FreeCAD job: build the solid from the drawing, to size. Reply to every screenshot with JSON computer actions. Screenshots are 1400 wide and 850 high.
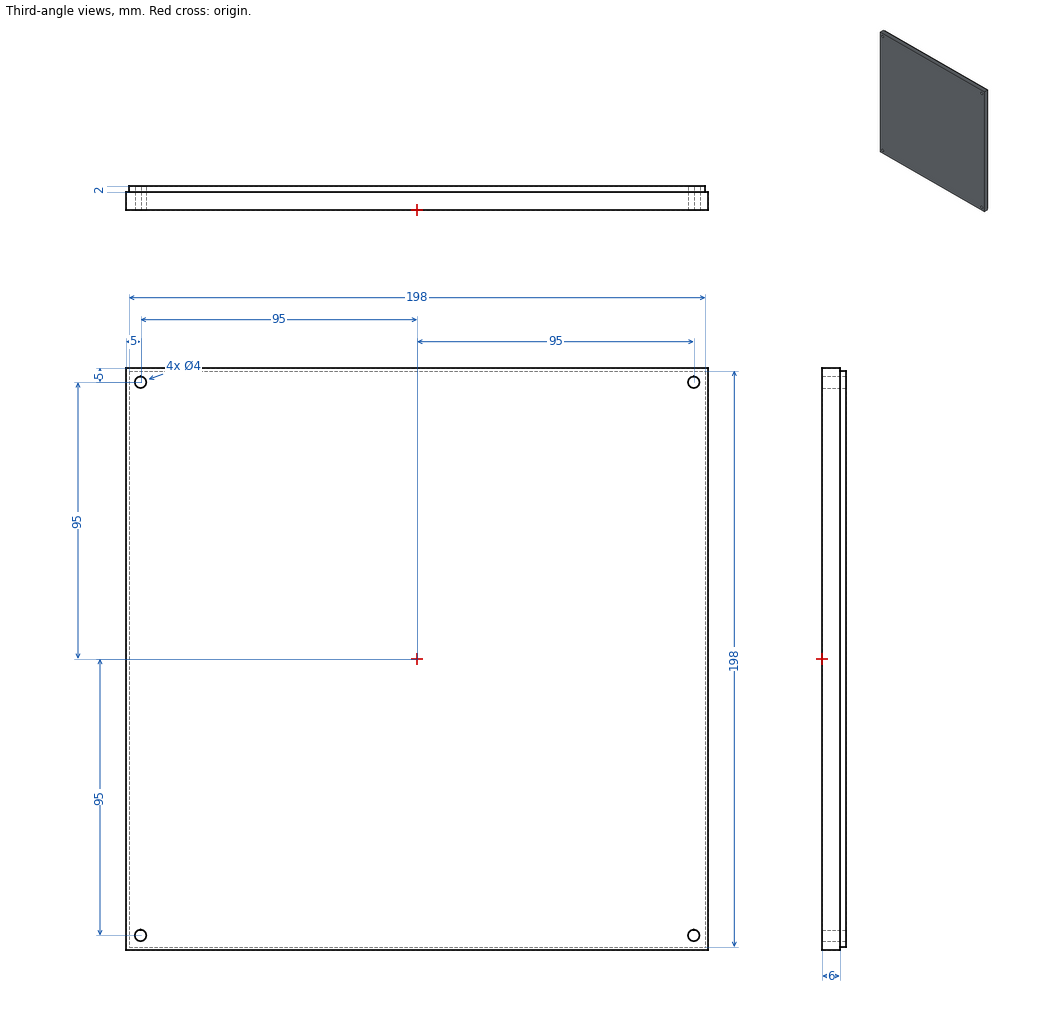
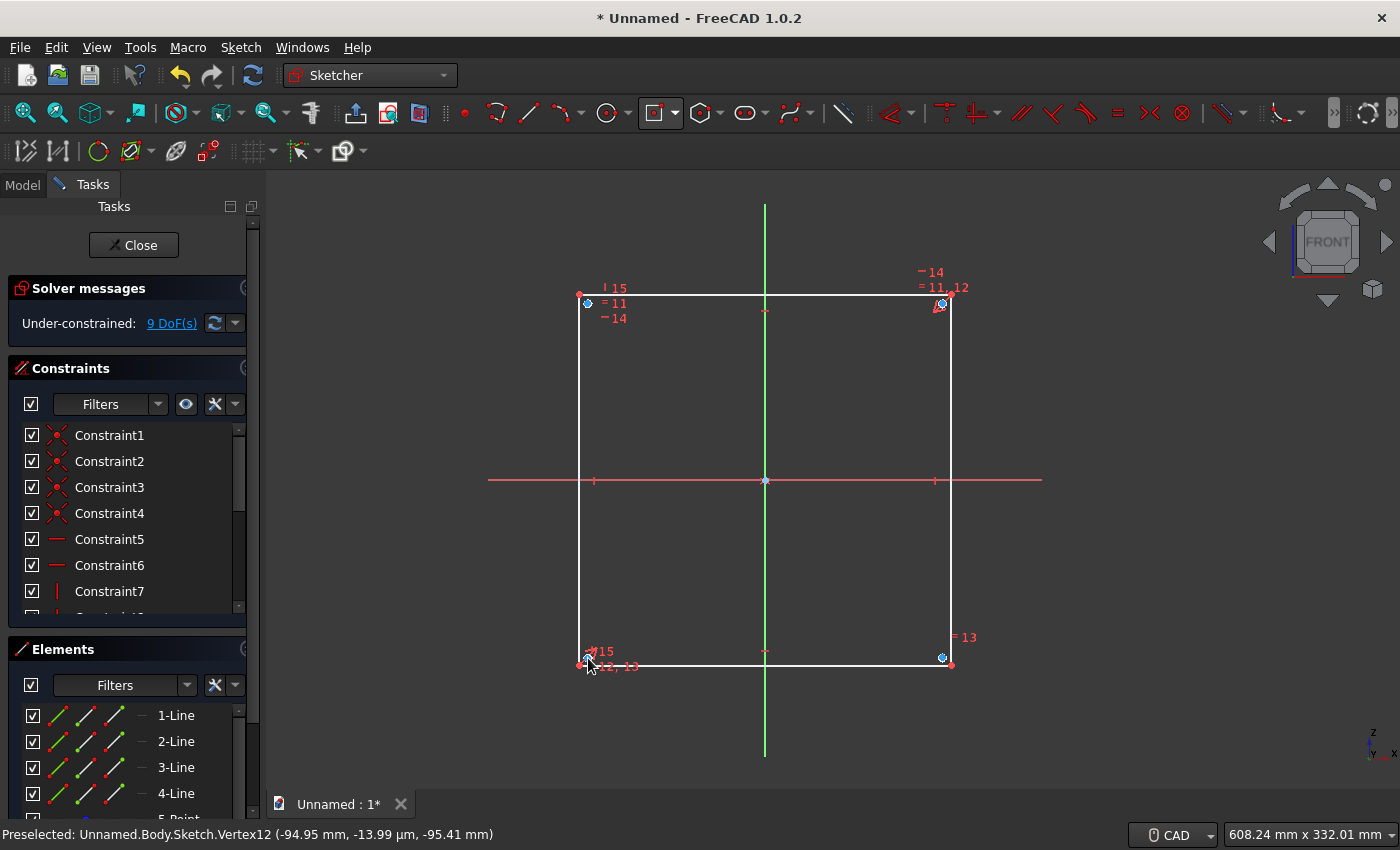
{"action": "left_click", "coordinate": [942, 304]}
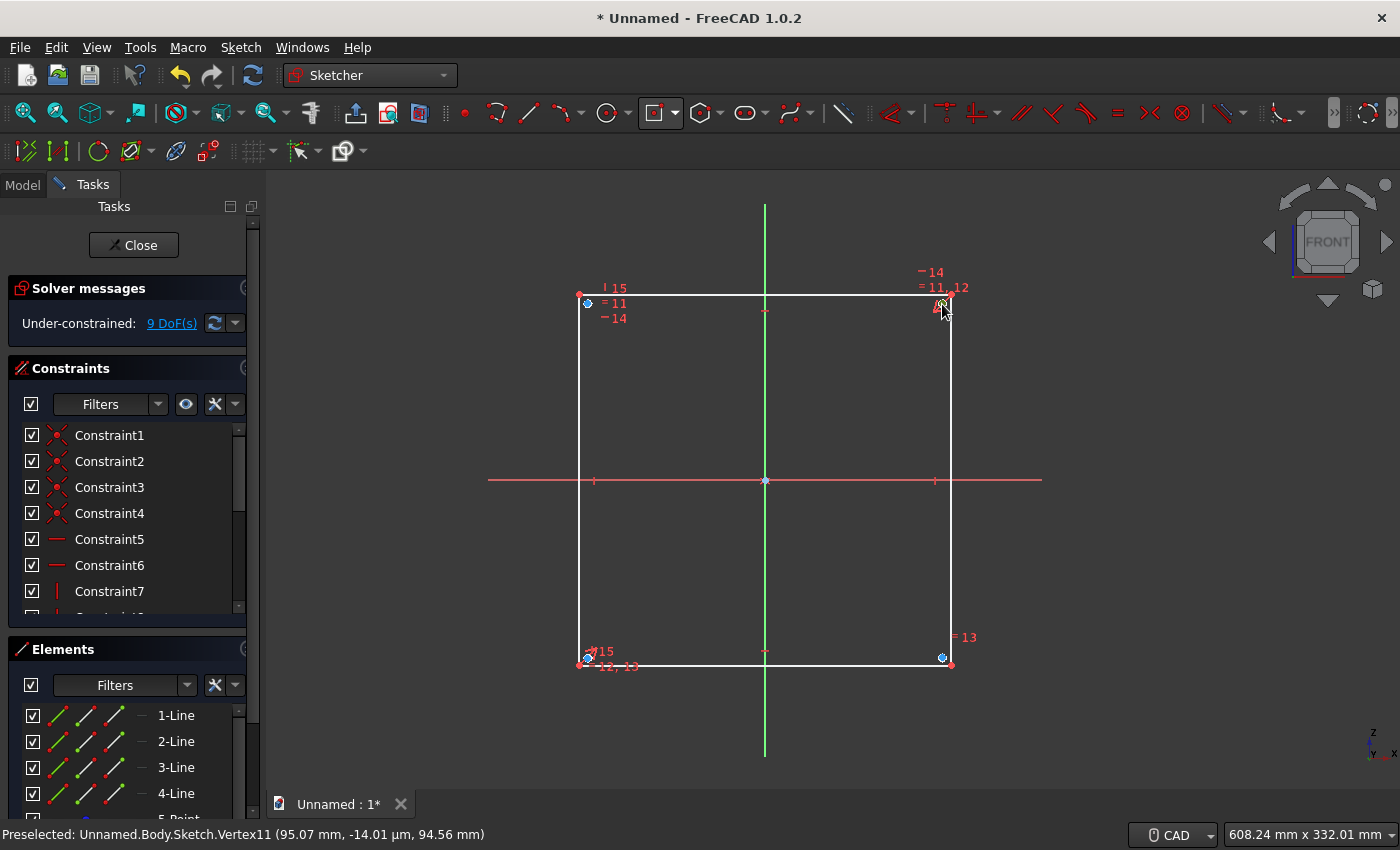
{"action": "left_click", "coordinate": [942, 658]}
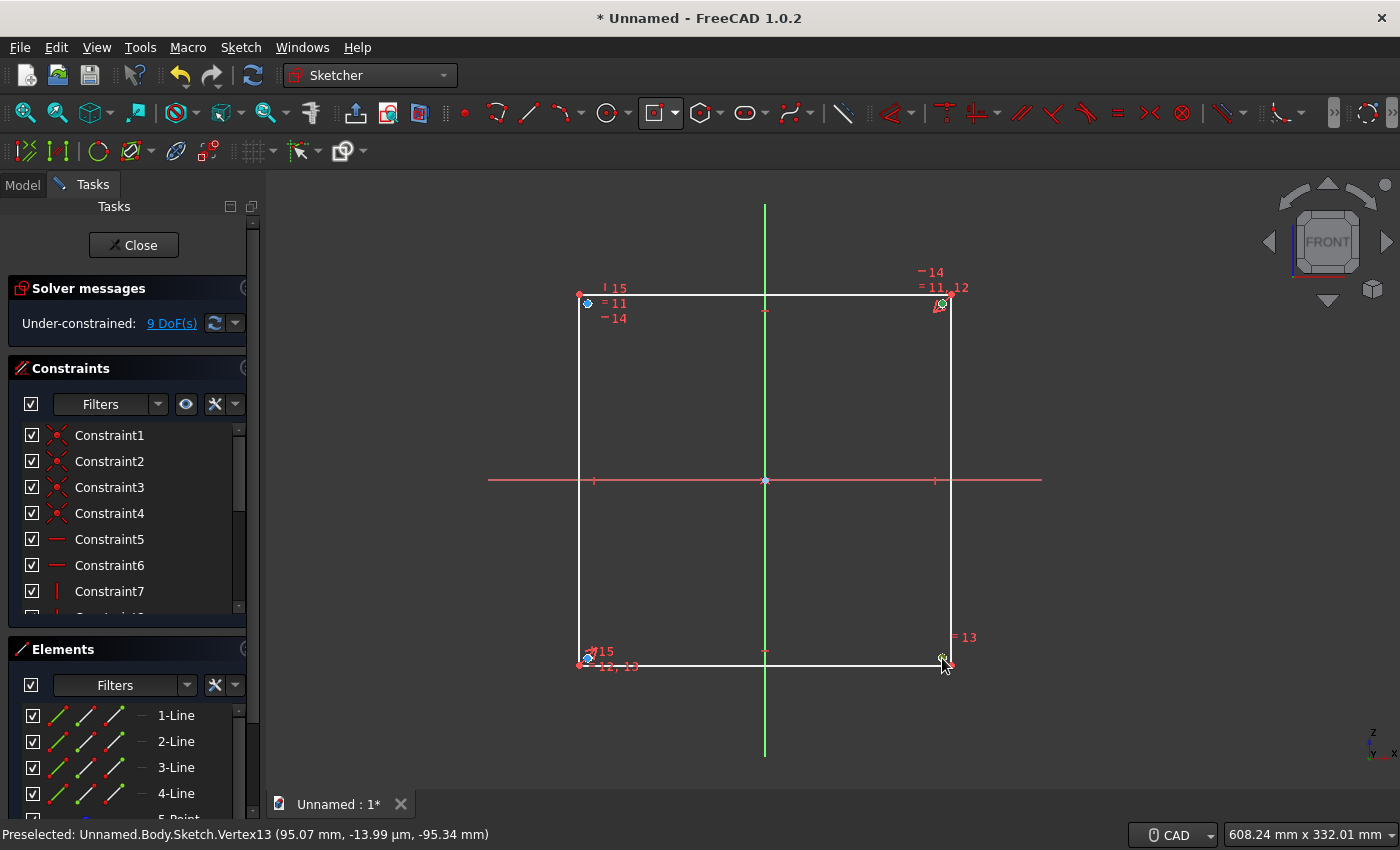
{"action": "key", "text": "v"}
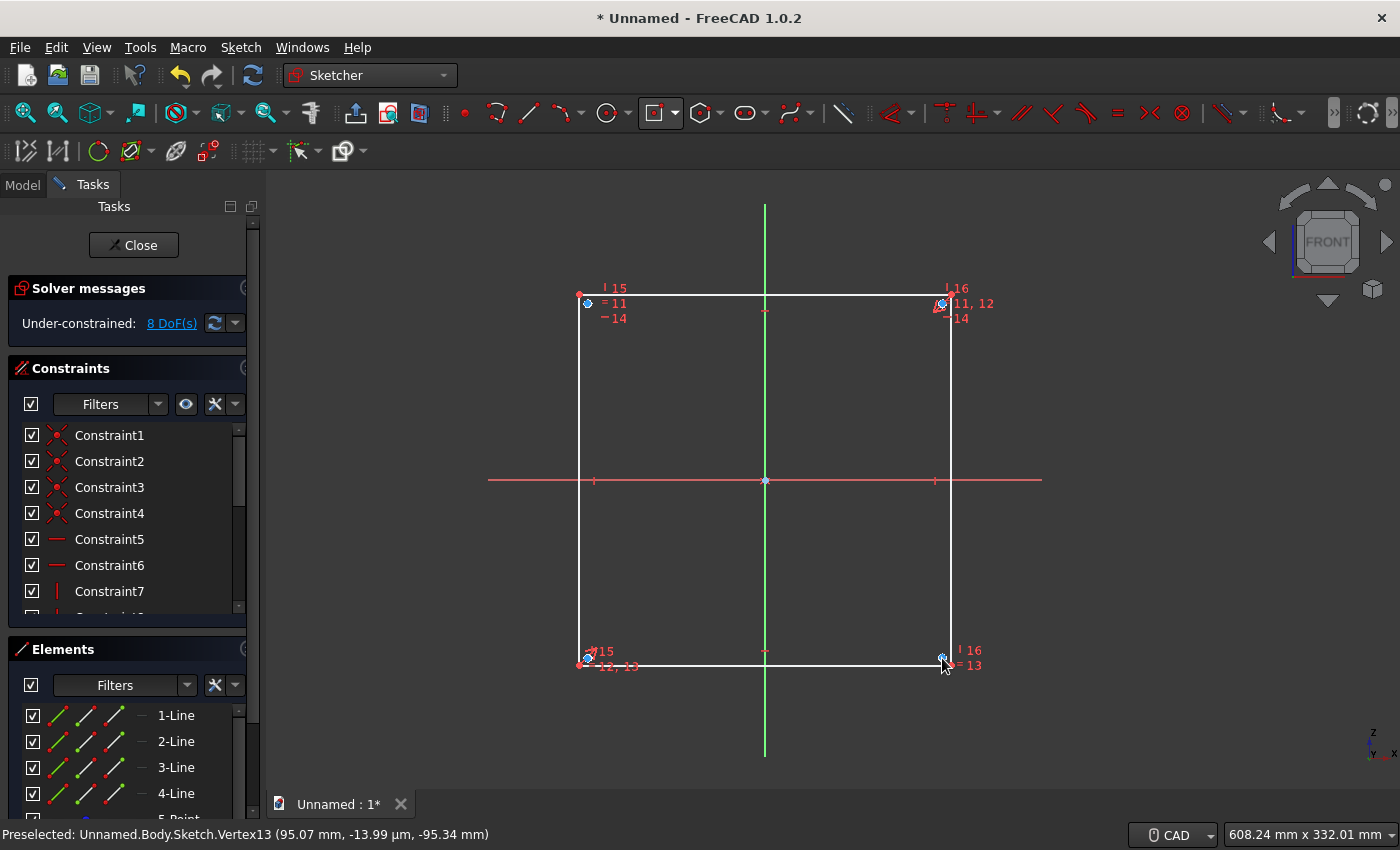
{"action": "left_click", "coordinate": [586, 660]}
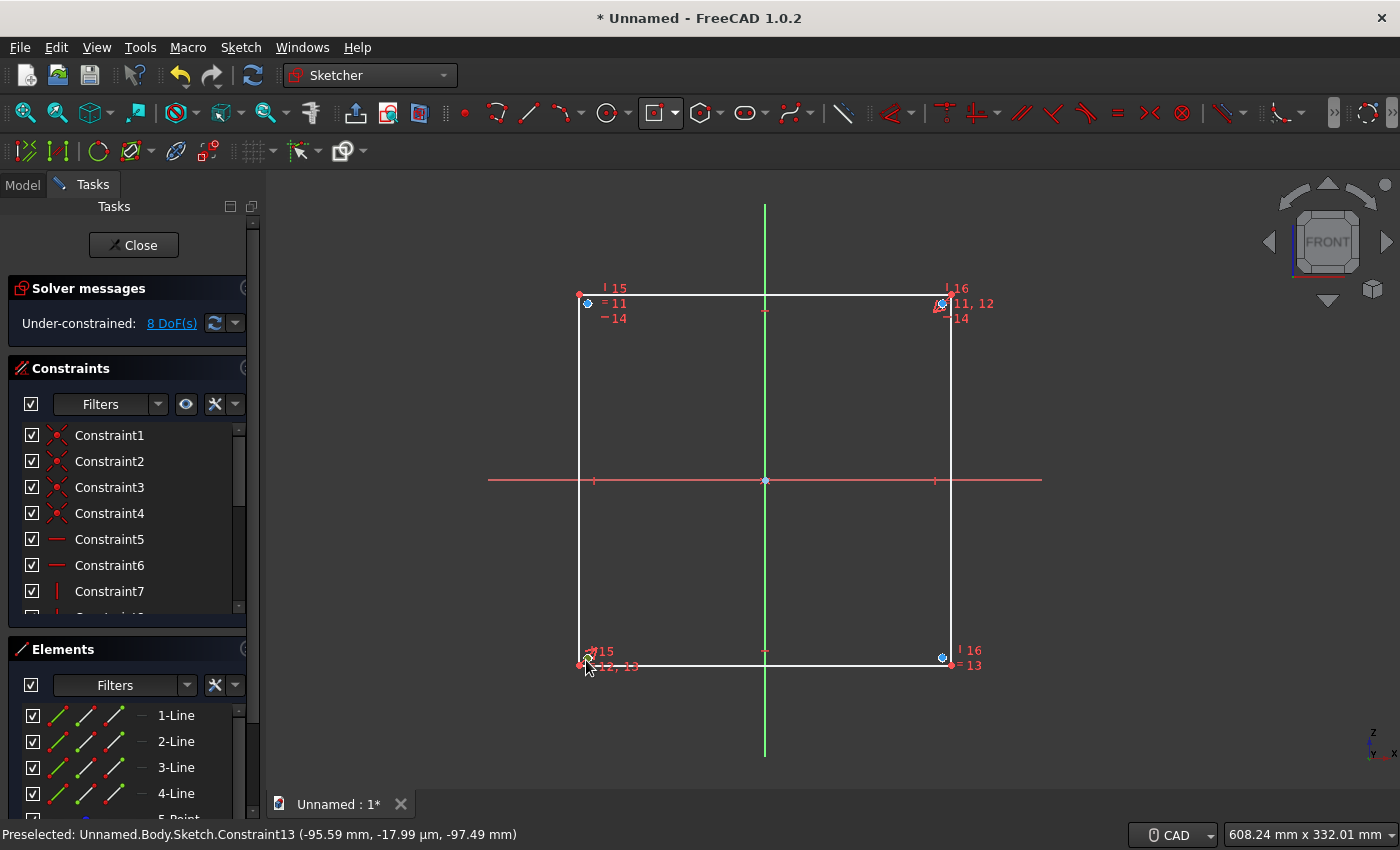
{"action": "left_click", "coordinate": [942, 658]}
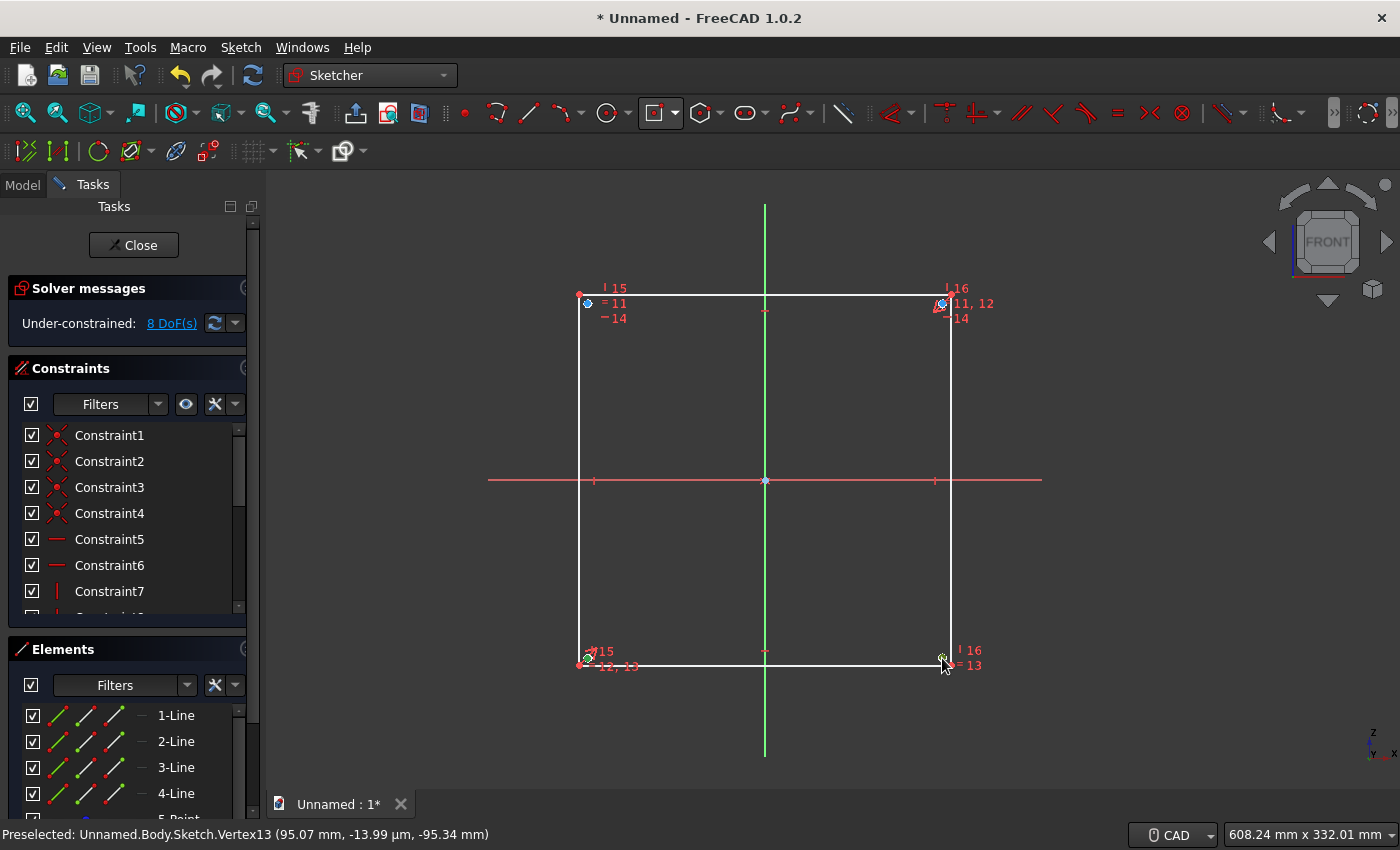
{"action": "left_click", "coordinate": [1000, 114]}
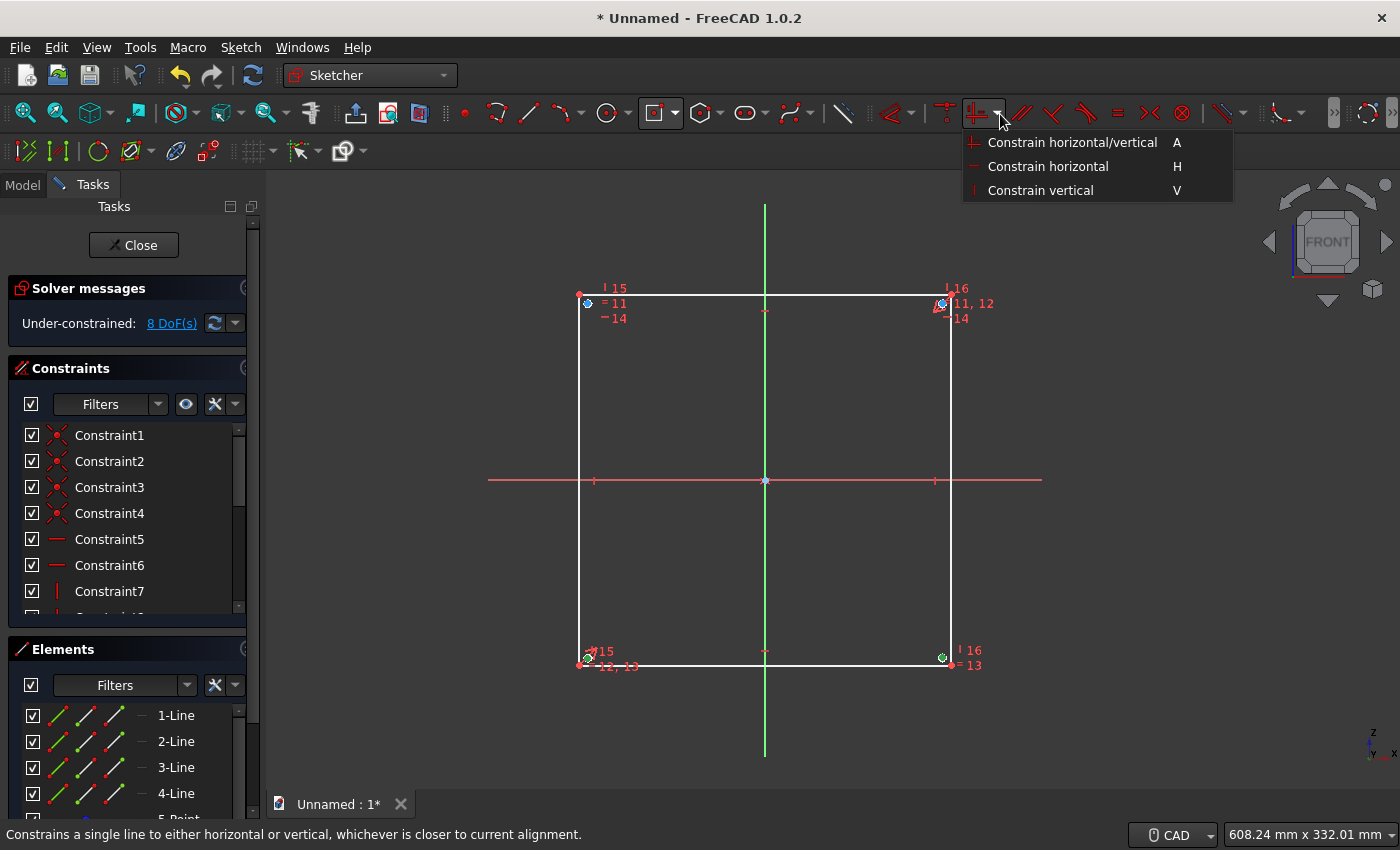
{"action": "left_click", "coordinate": [1098, 166]}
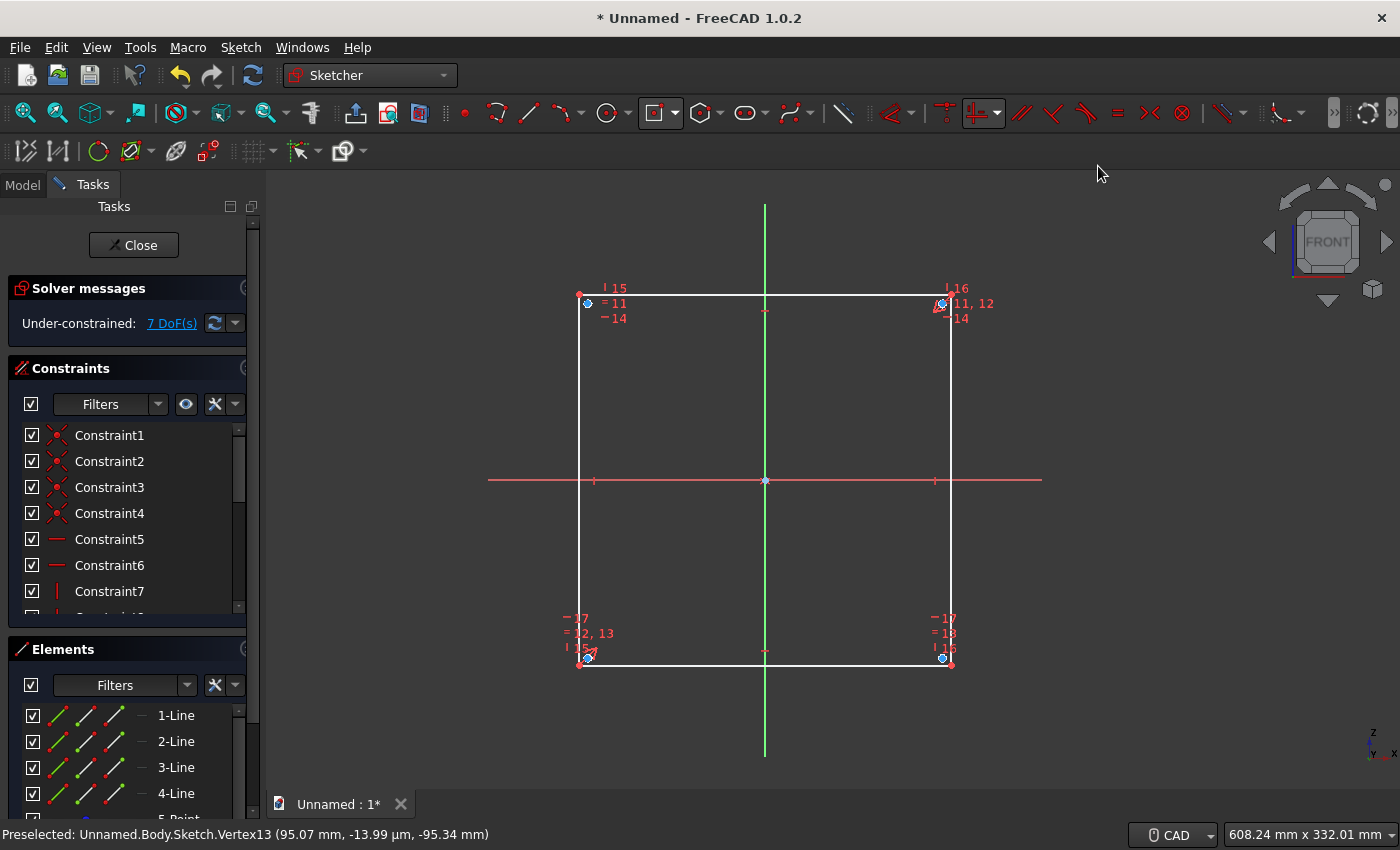
{"action": "left_click", "coordinate": [890, 114]}